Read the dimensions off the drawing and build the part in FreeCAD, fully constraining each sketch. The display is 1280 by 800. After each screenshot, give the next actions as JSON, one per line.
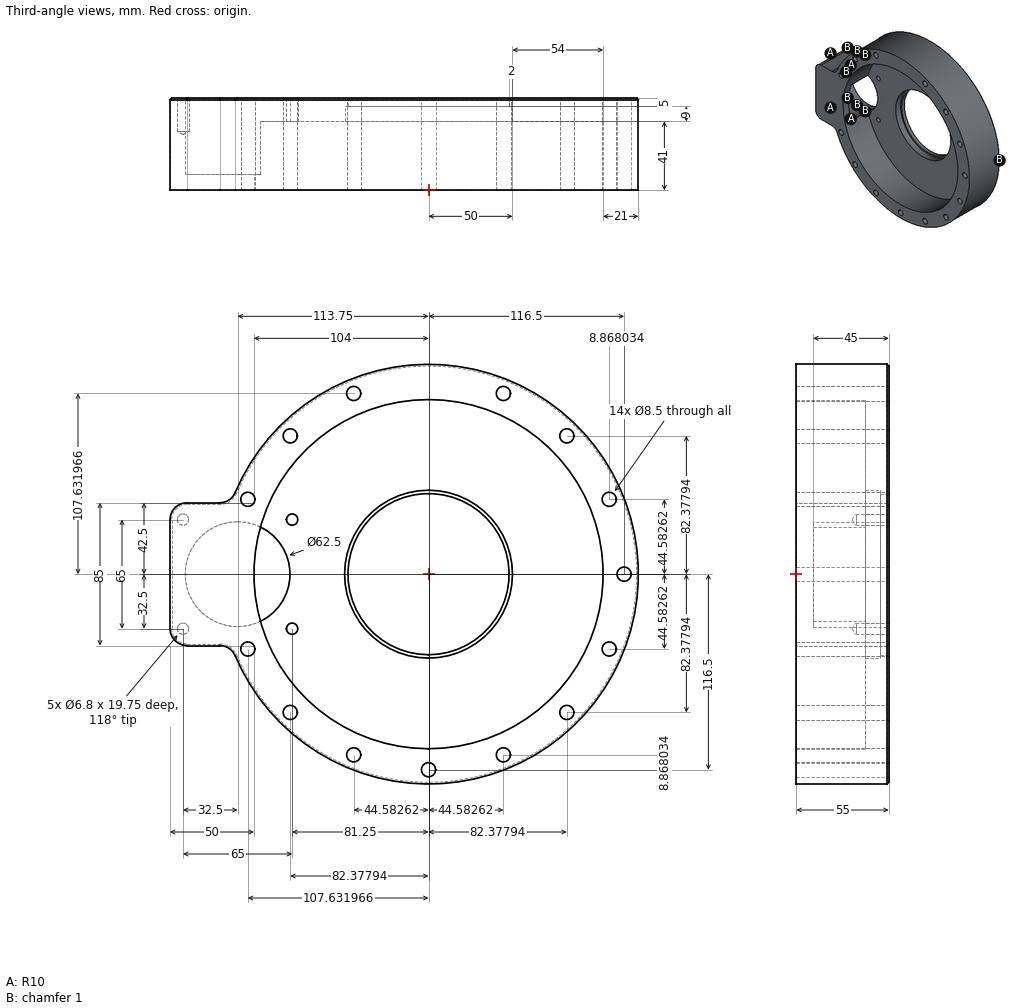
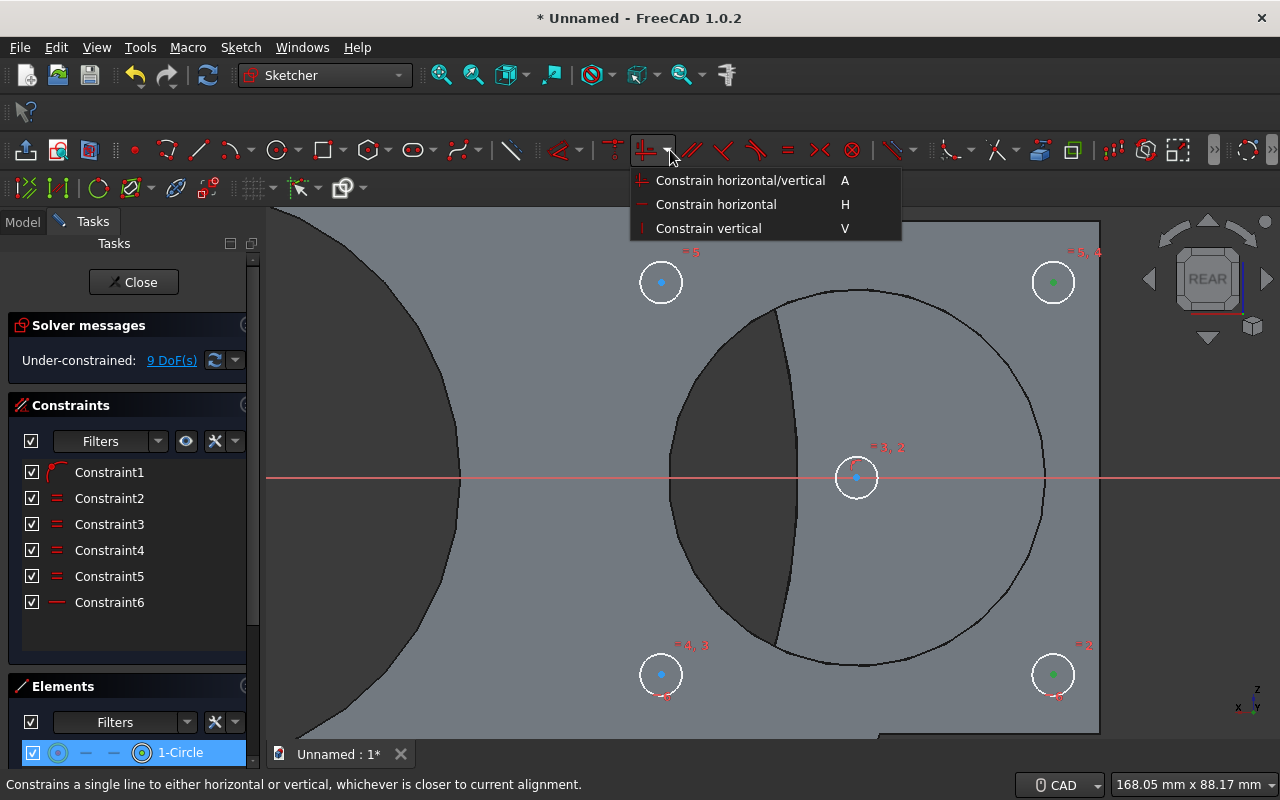
{"action": "left_click", "coordinate": [766, 228]}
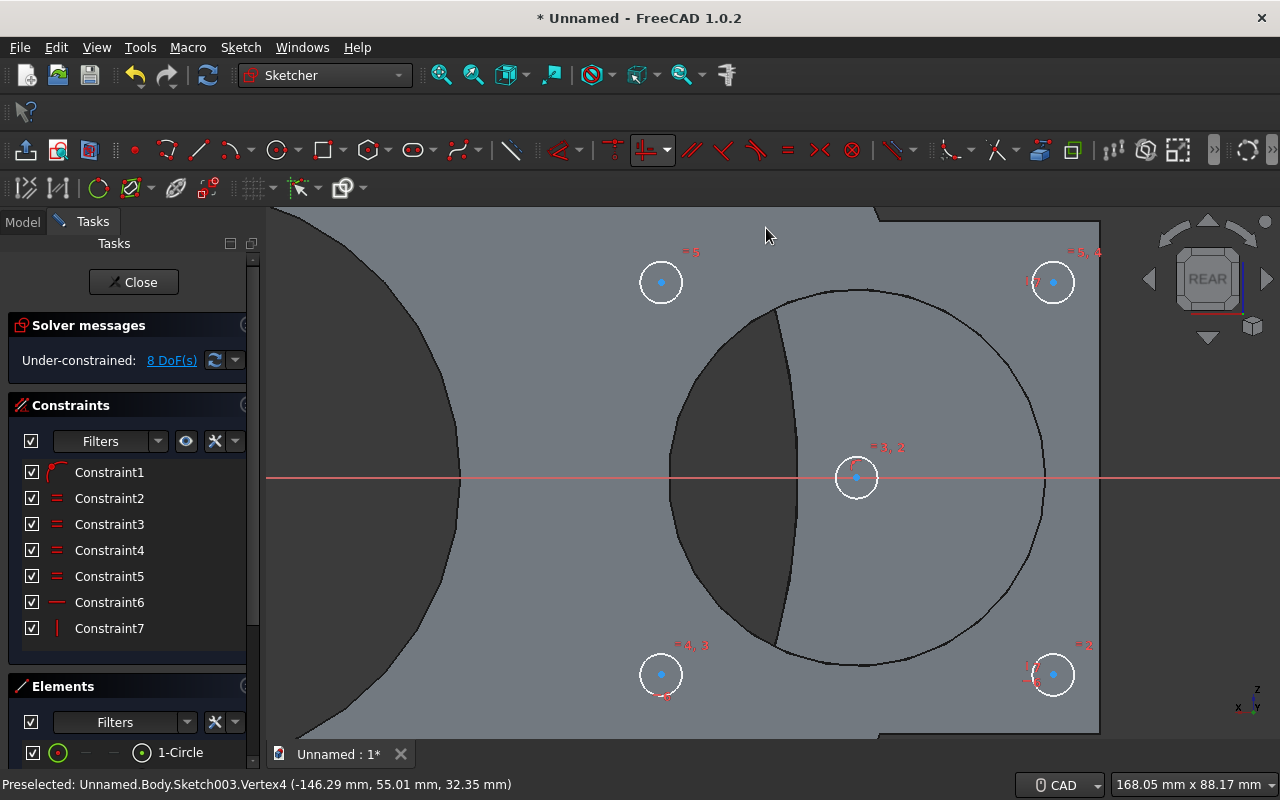
{"action": "left_click", "coordinate": [661, 675]}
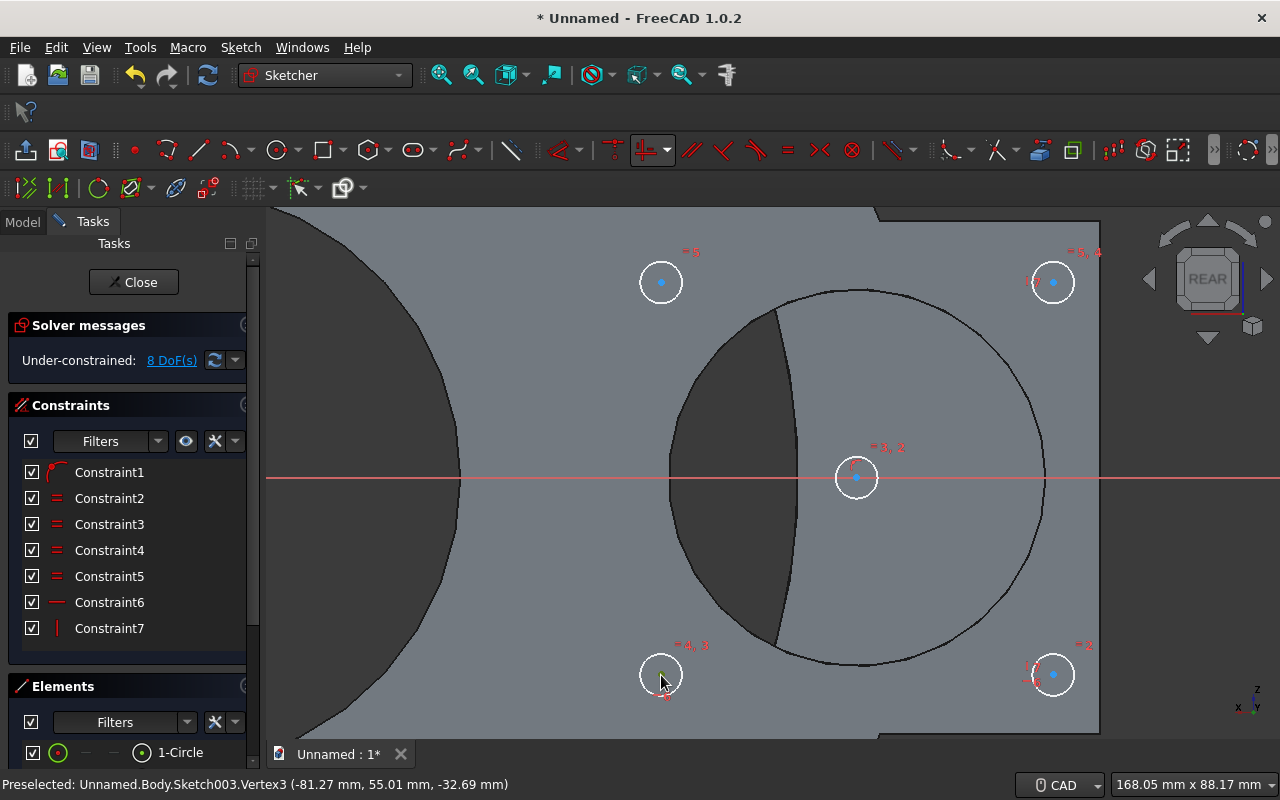
{"action": "left_click", "coordinate": [661, 283]}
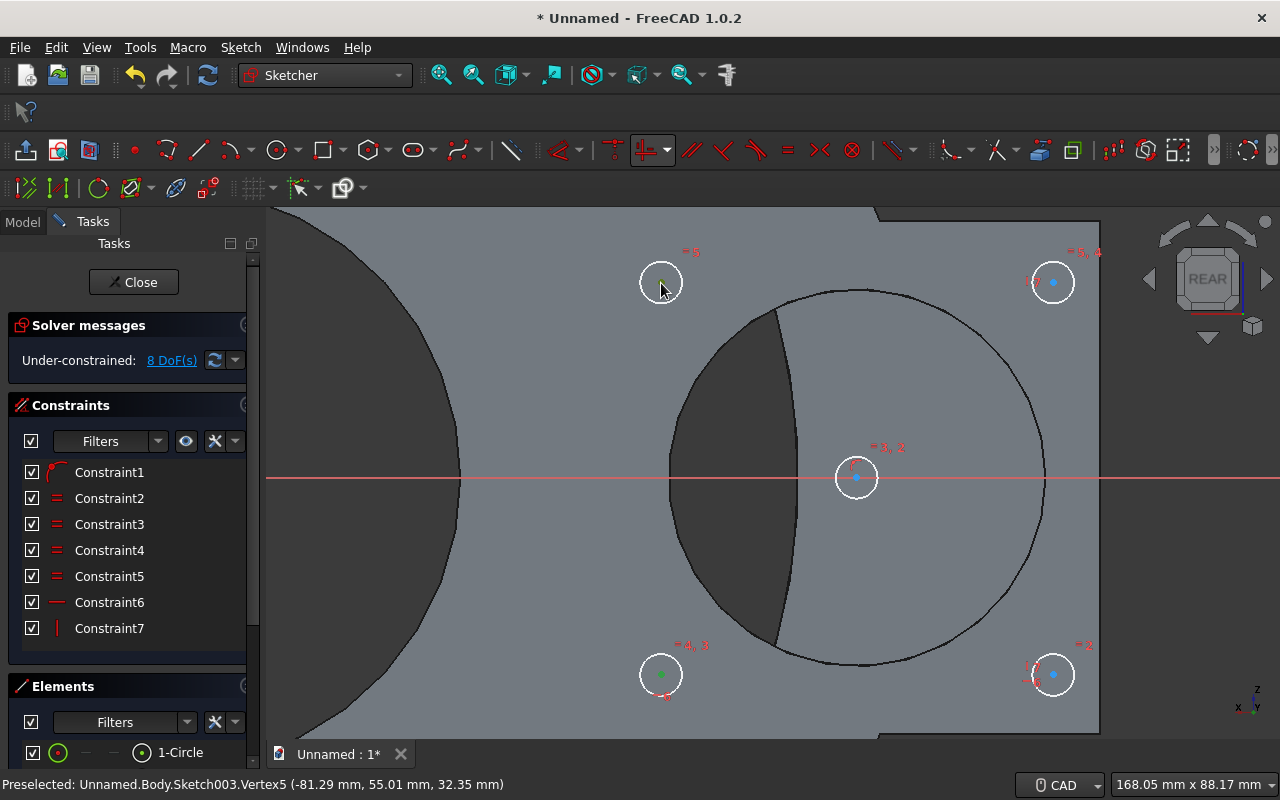
{"action": "left_click", "coordinate": [670, 150]}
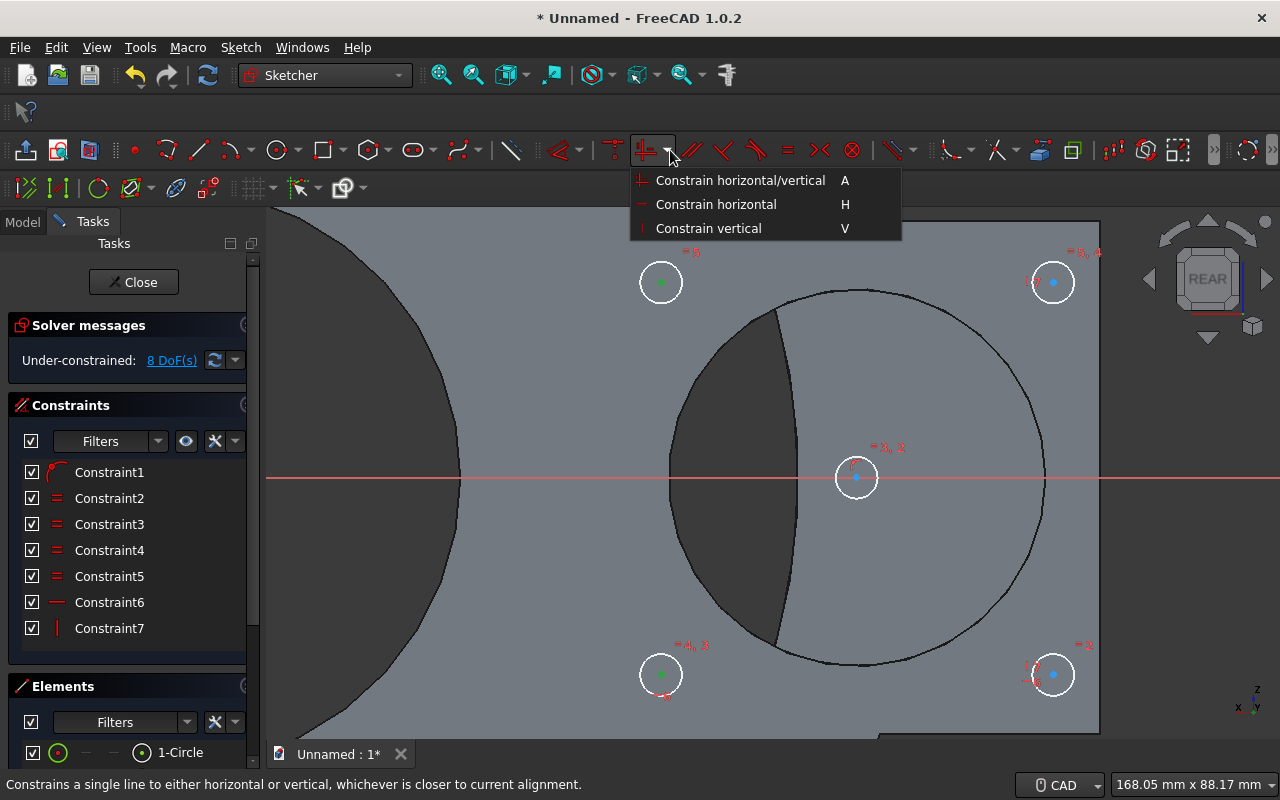
{"action": "left_click", "coordinate": [766, 228]}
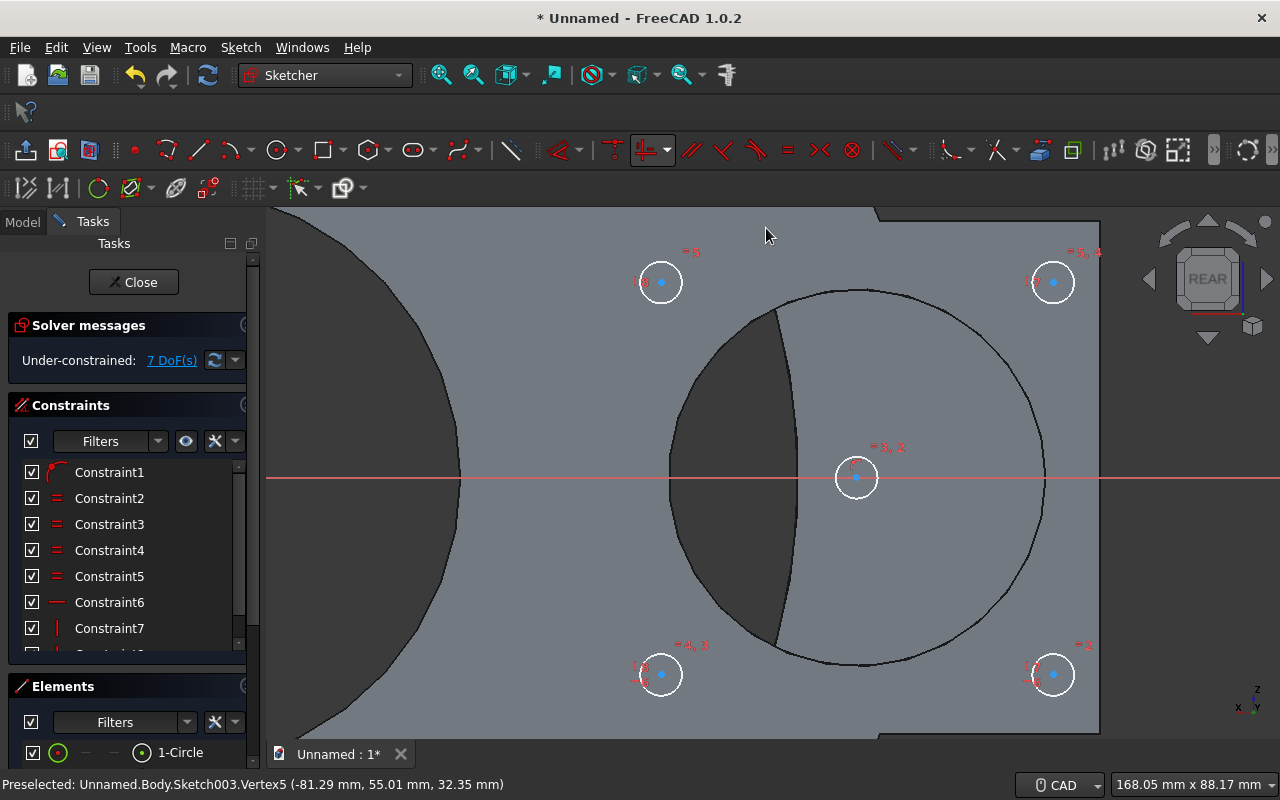
{"action": "left_click", "coordinate": [1053, 283]}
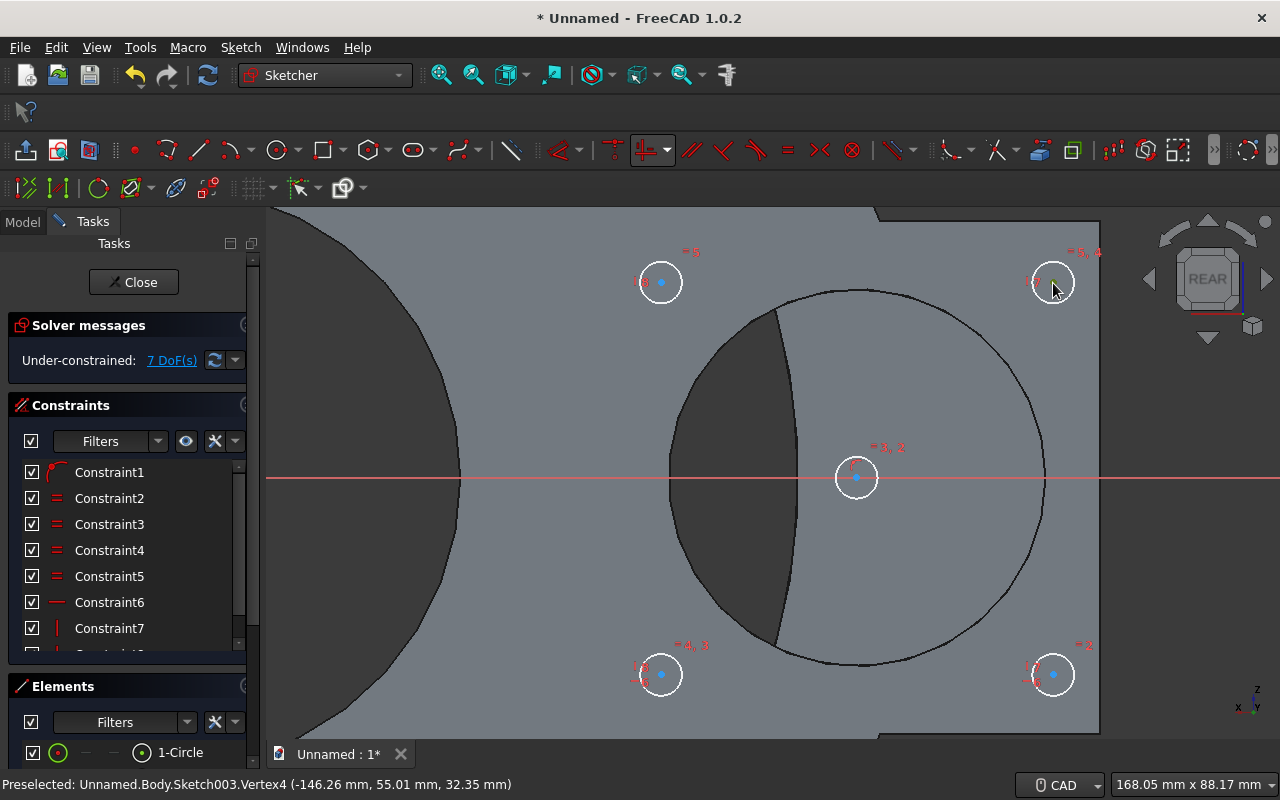
{"action": "left_click", "coordinate": [661, 283]}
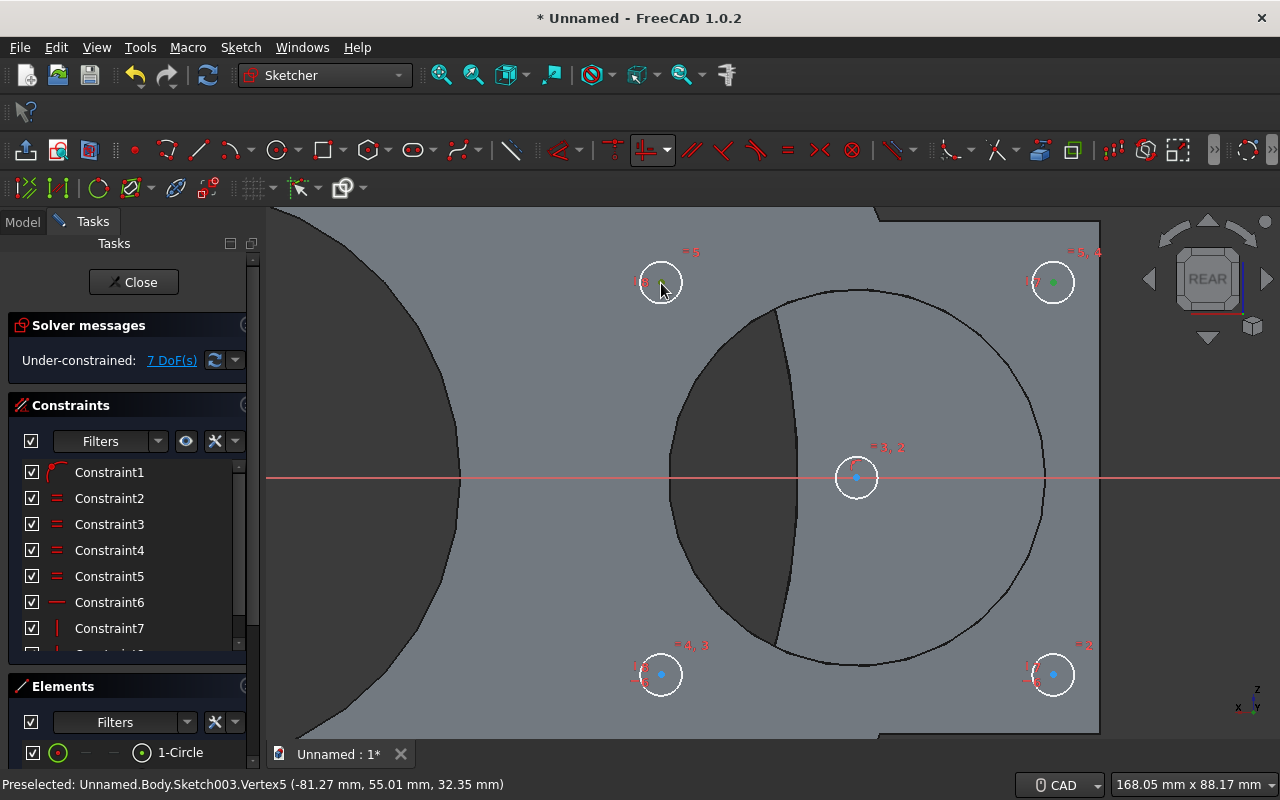
{"action": "key", "text": "h"}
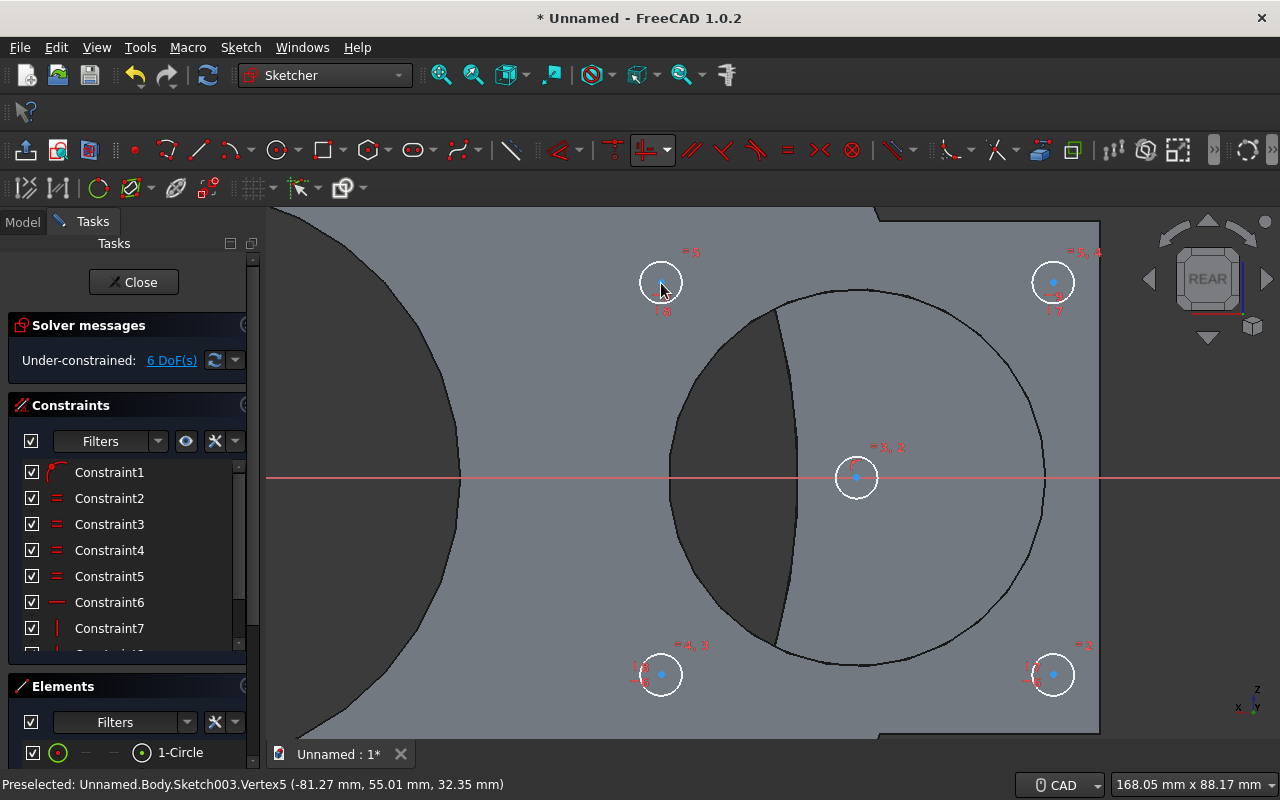
{"action": "left_click", "coordinate": [558, 150]}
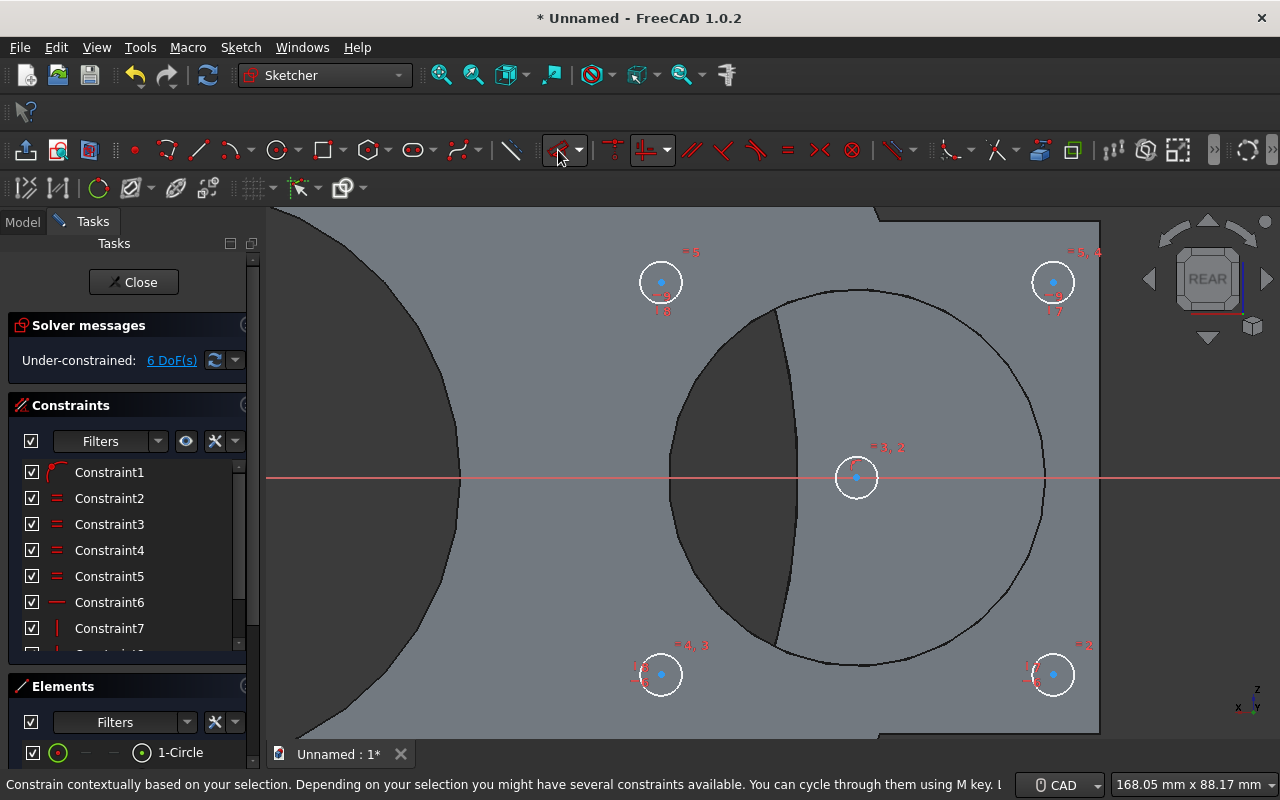
{"action": "left_click", "coordinate": [1068, 660]}
{"action": "left_click", "coordinate": [1090, 637]}